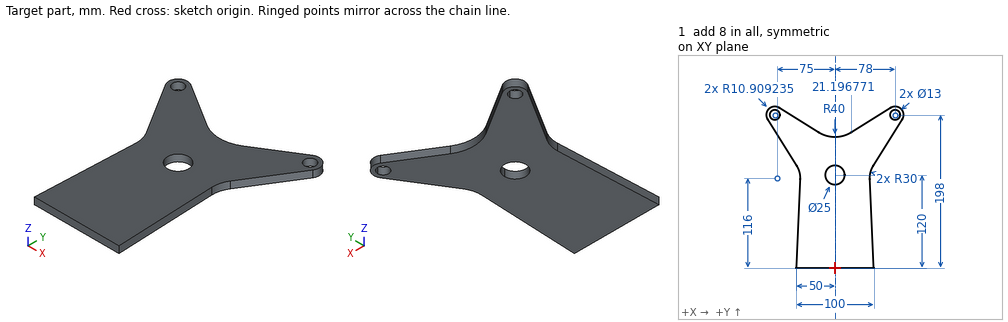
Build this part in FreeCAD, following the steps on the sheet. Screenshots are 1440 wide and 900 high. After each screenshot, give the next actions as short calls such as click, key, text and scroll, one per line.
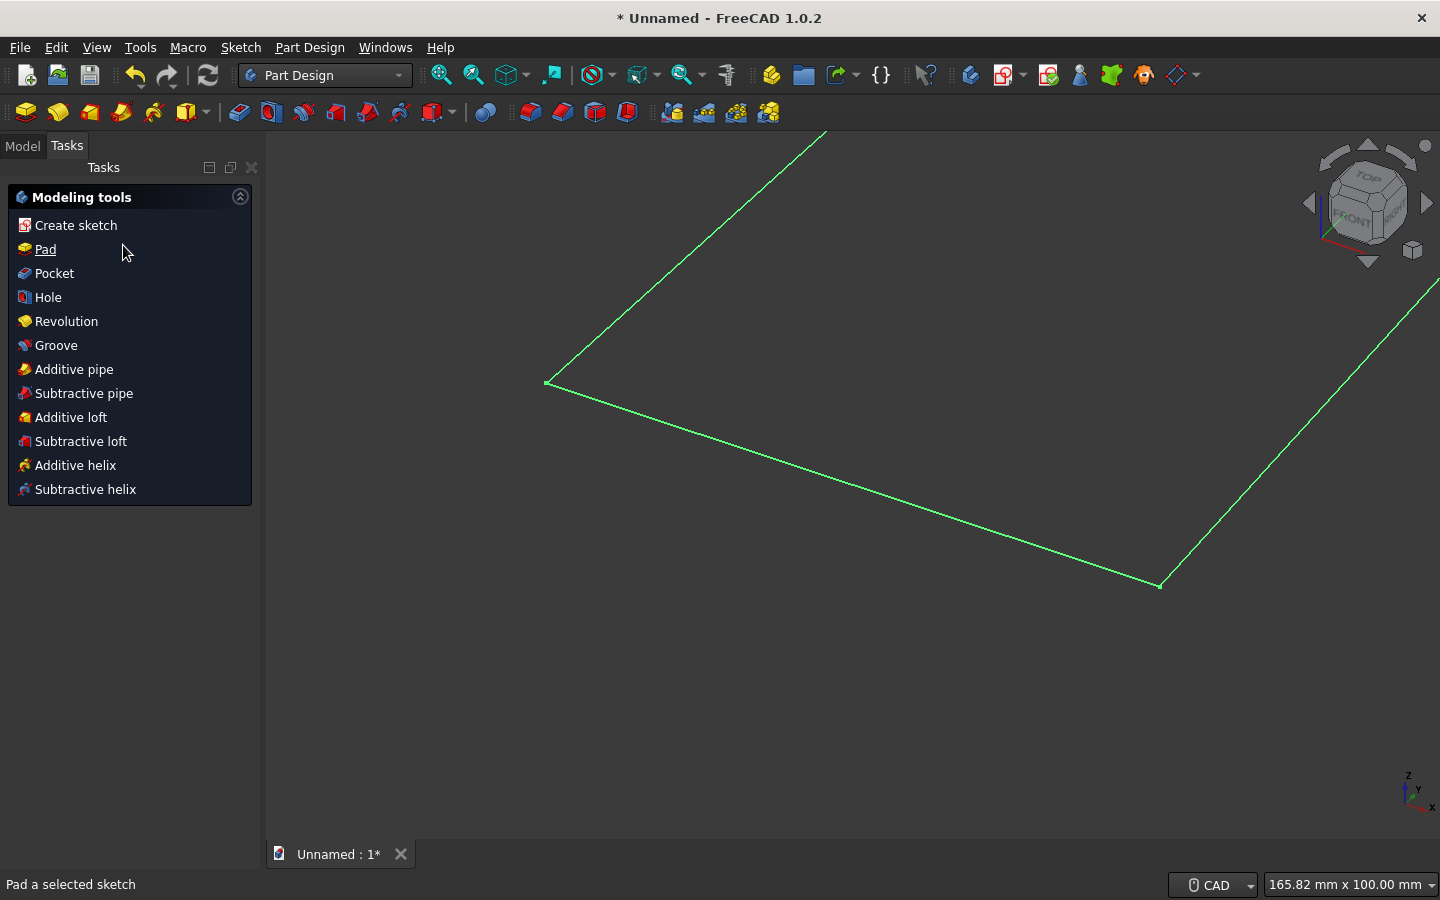
click(26, 112)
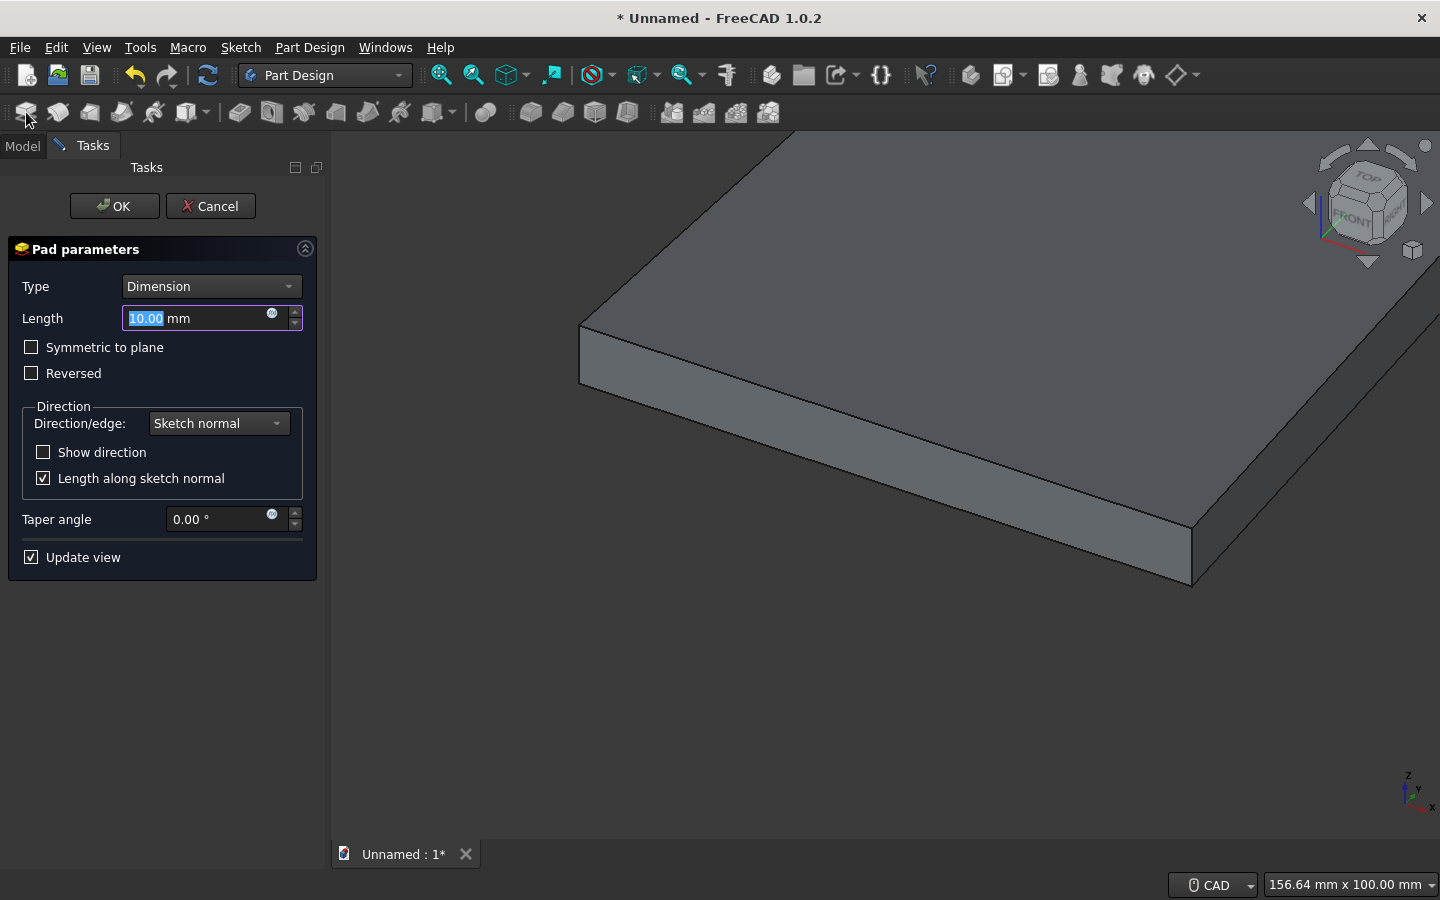
text(8)
key(Tab)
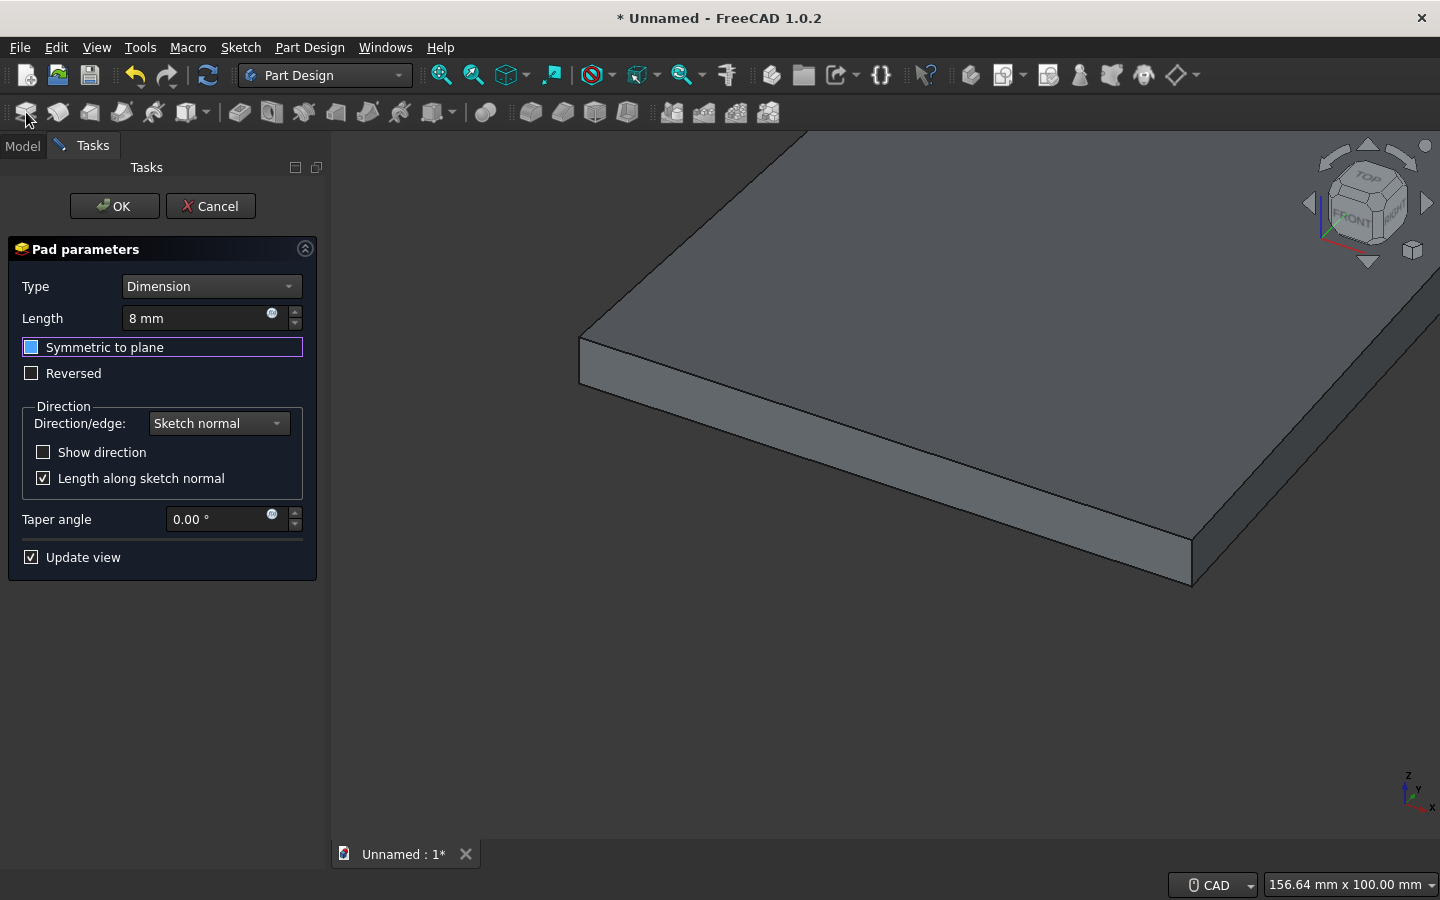
click(30, 347)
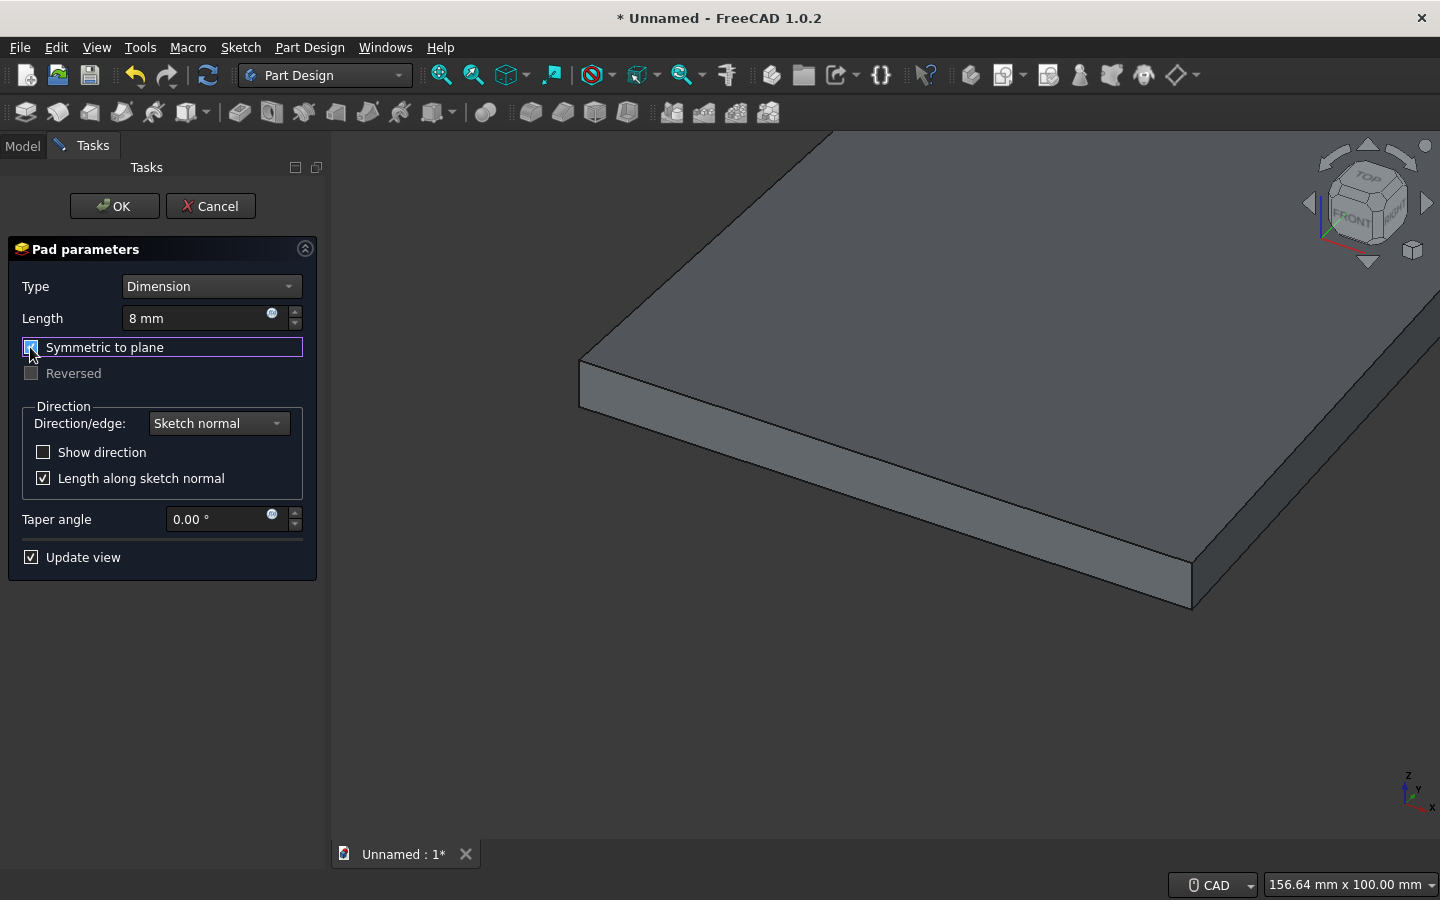
click(115, 206)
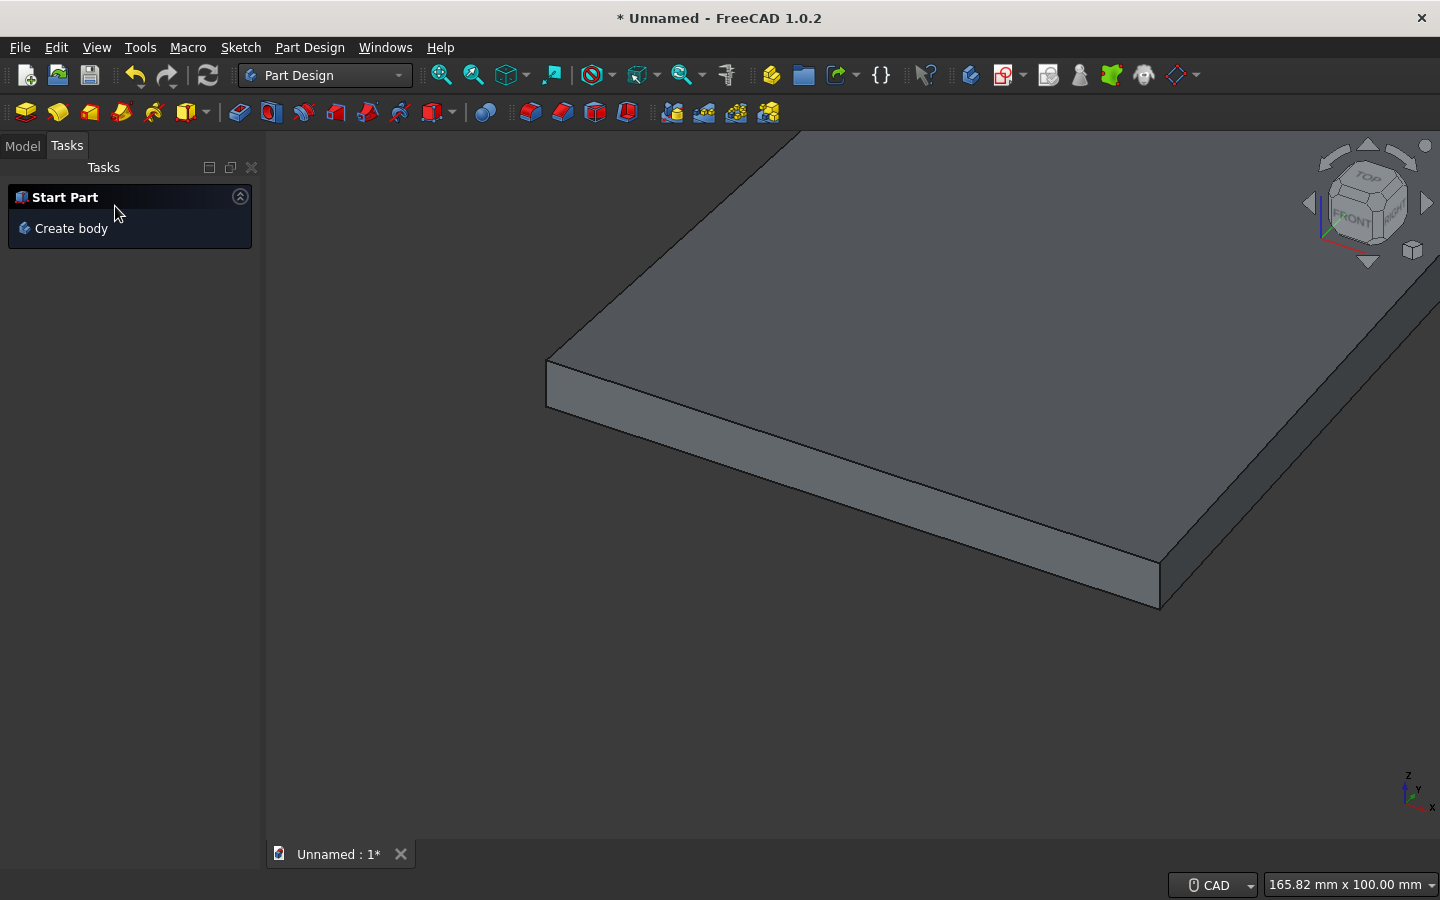
key(0)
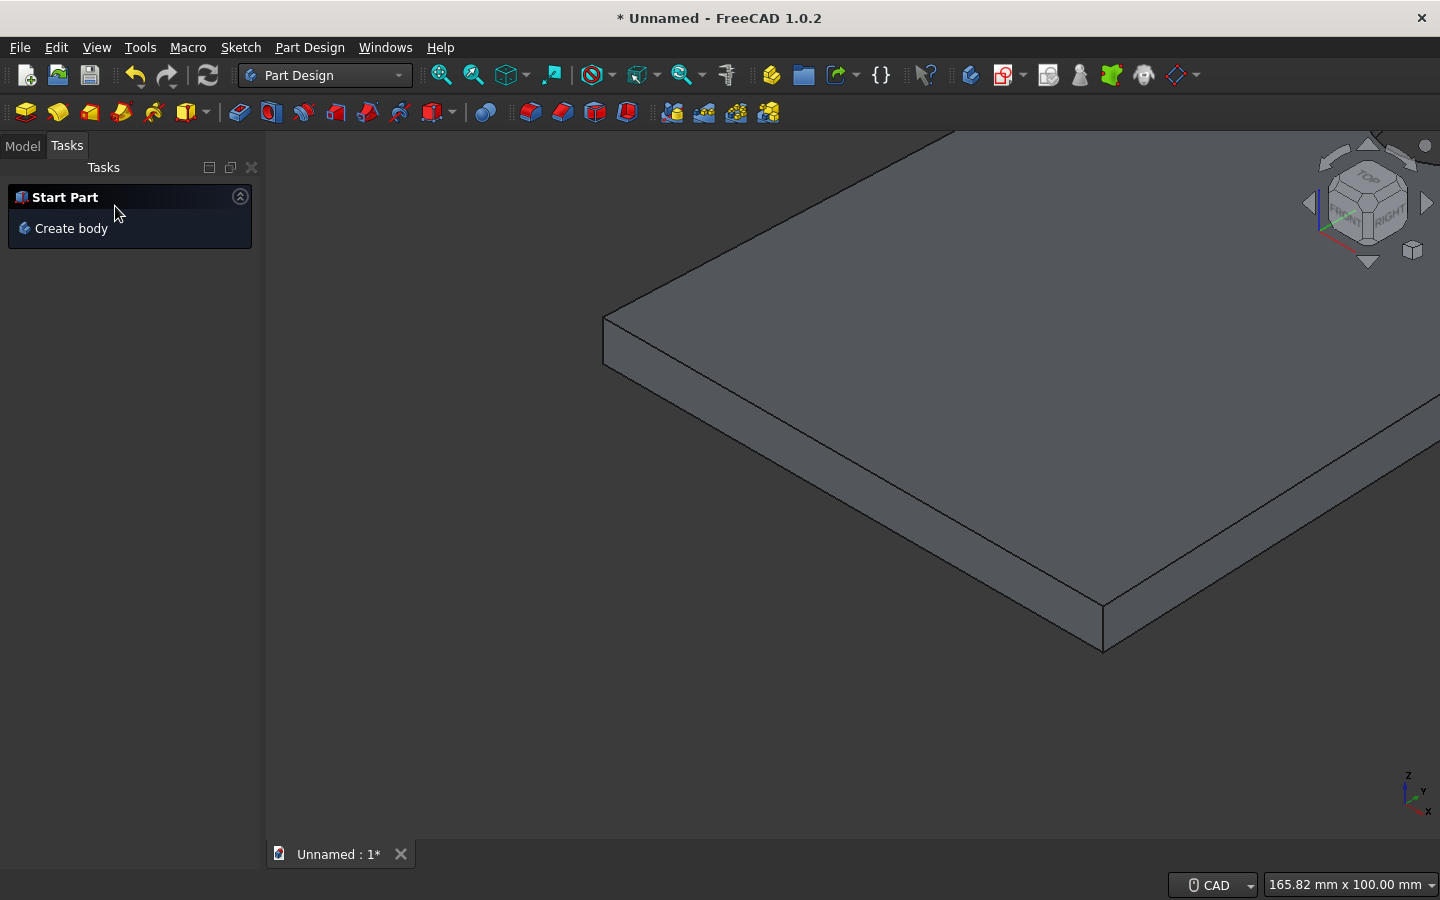
click(442, 76)